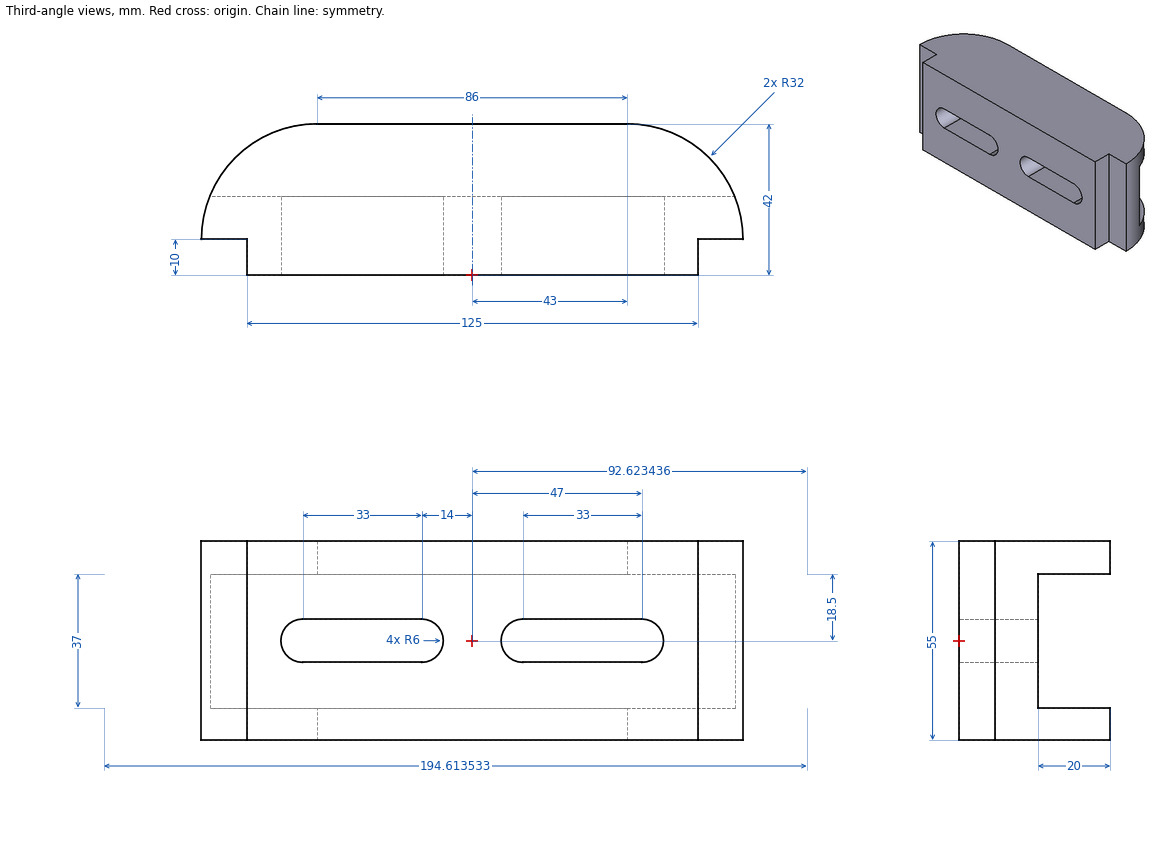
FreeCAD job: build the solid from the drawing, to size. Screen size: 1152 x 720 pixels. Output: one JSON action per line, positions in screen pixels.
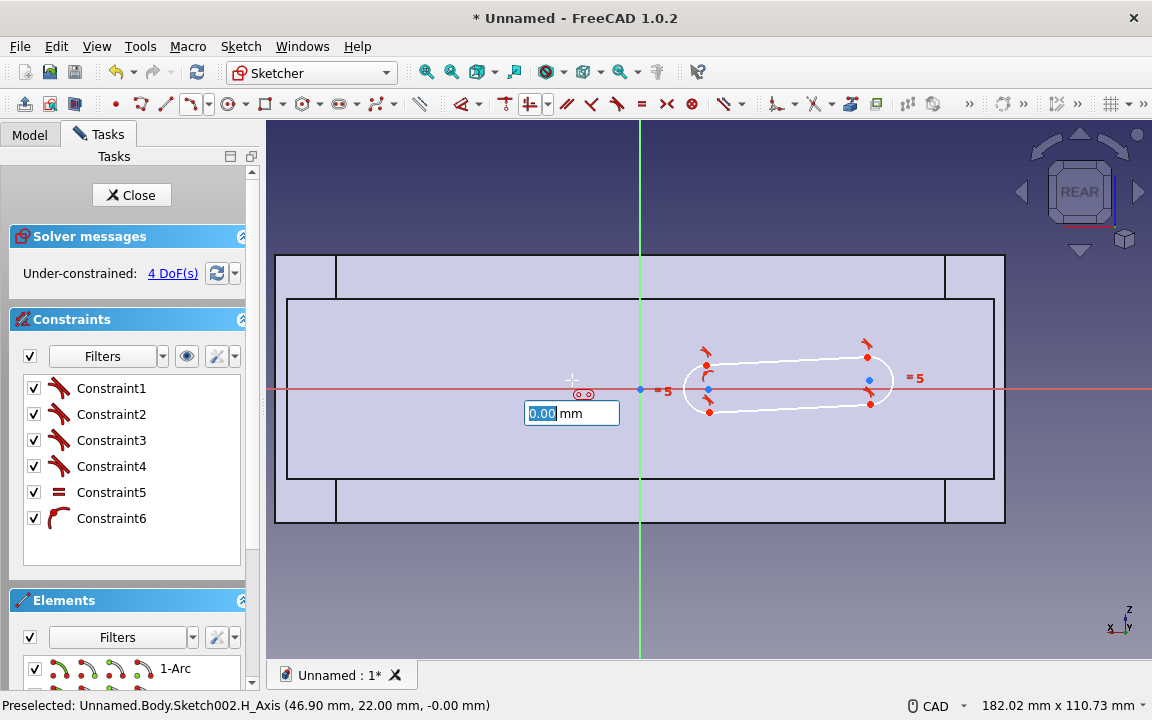
{"action": "left_click", "coordinate": [492, 418]}
{"action": "key", "text": "Escape"}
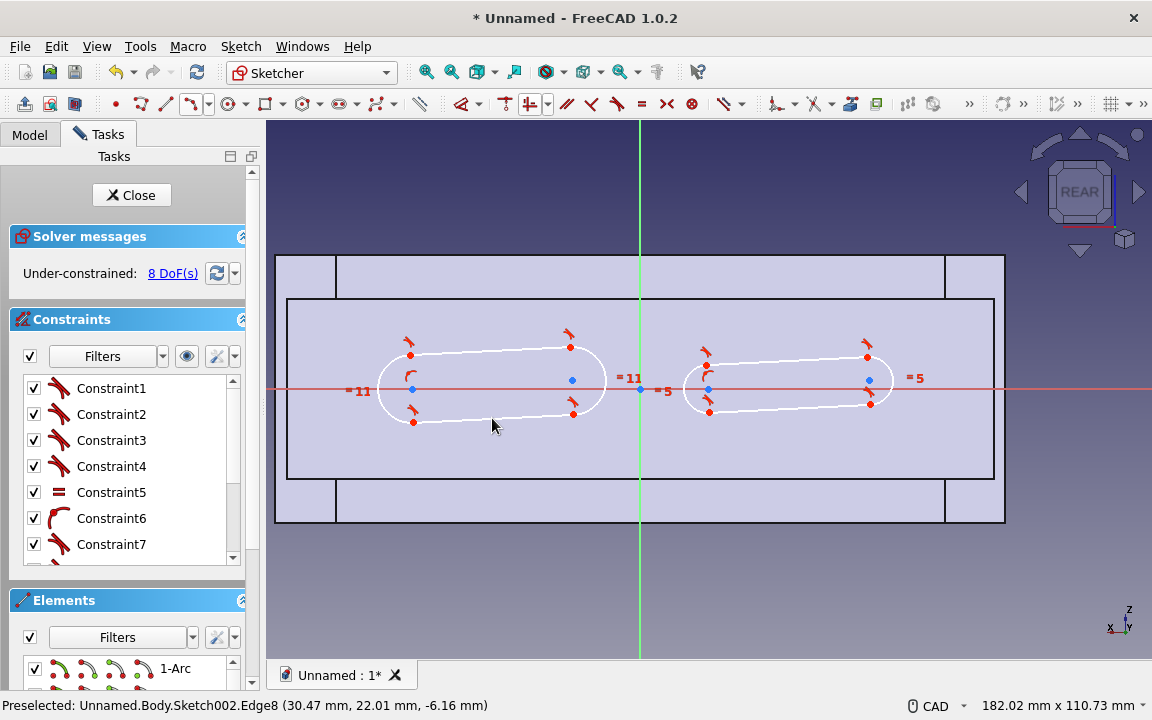
{"action": "left_click", "coordinate": [755, 363]}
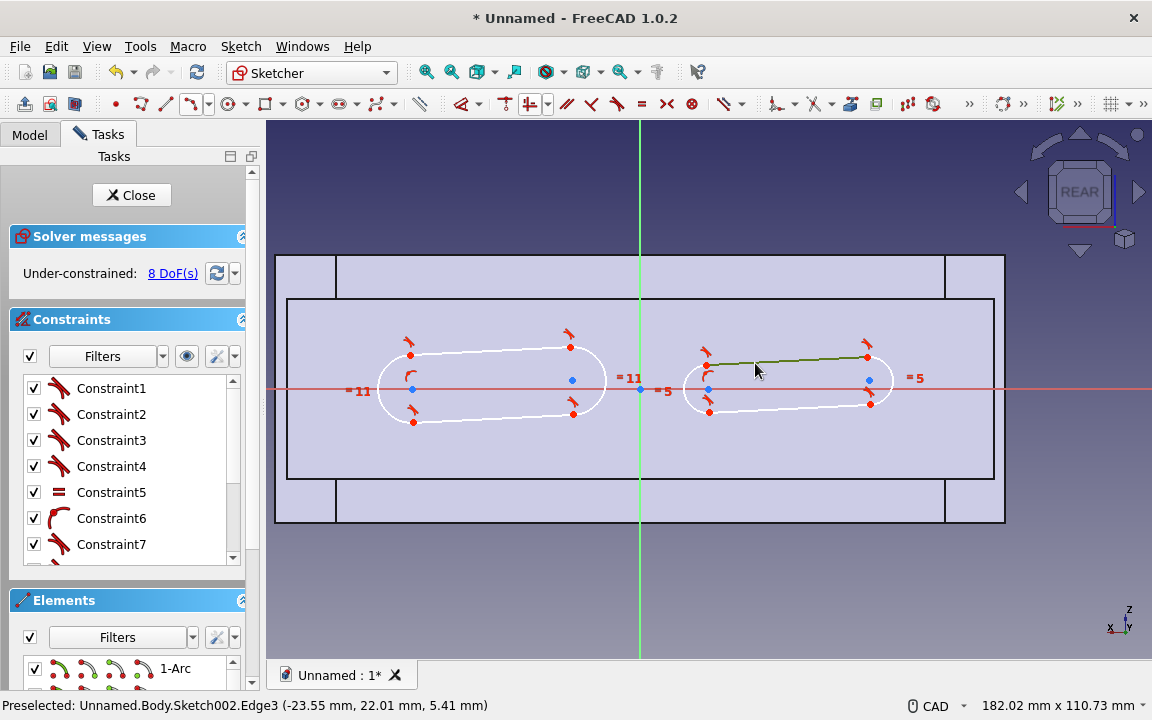
{"action": "key", "text": "h"}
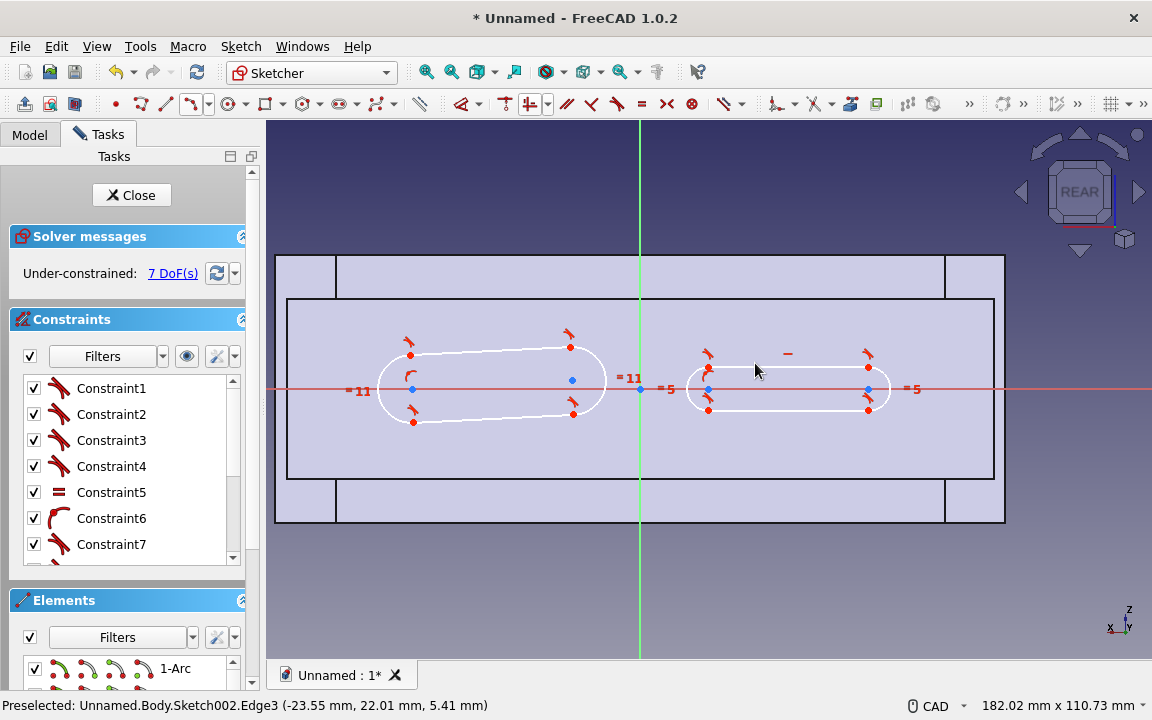
{"action": "left_click", "coordinate": [458, 353]}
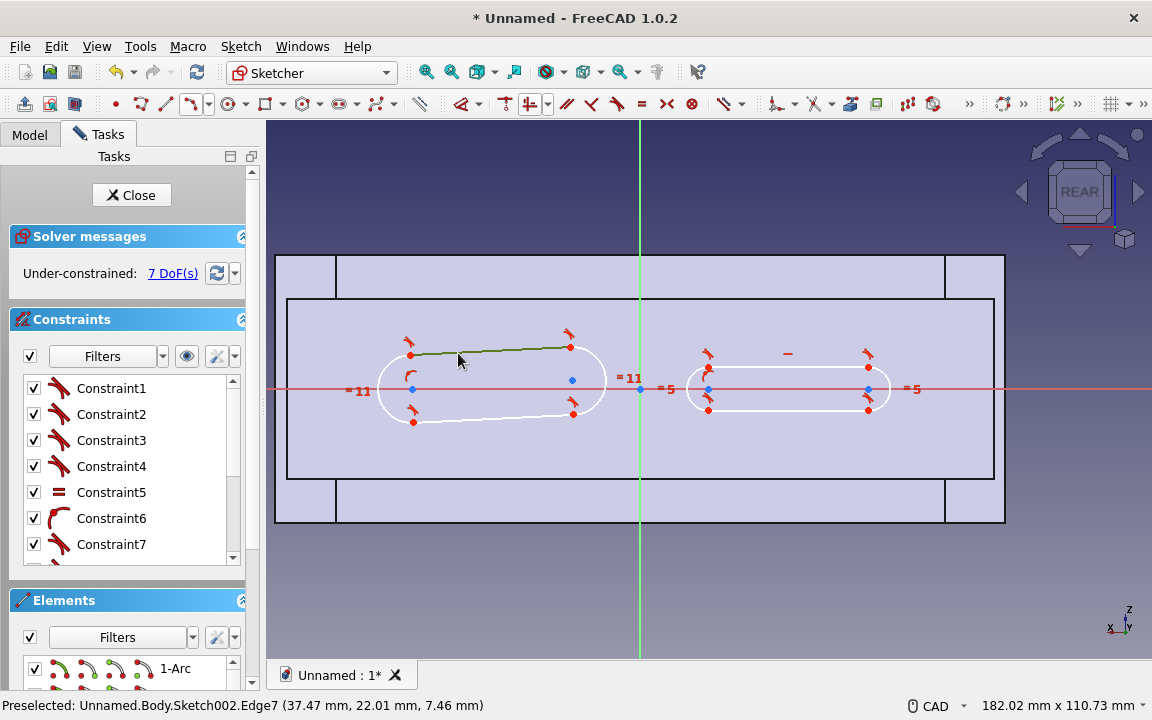
{"action": "left_click", "coordinate": [548, 104]}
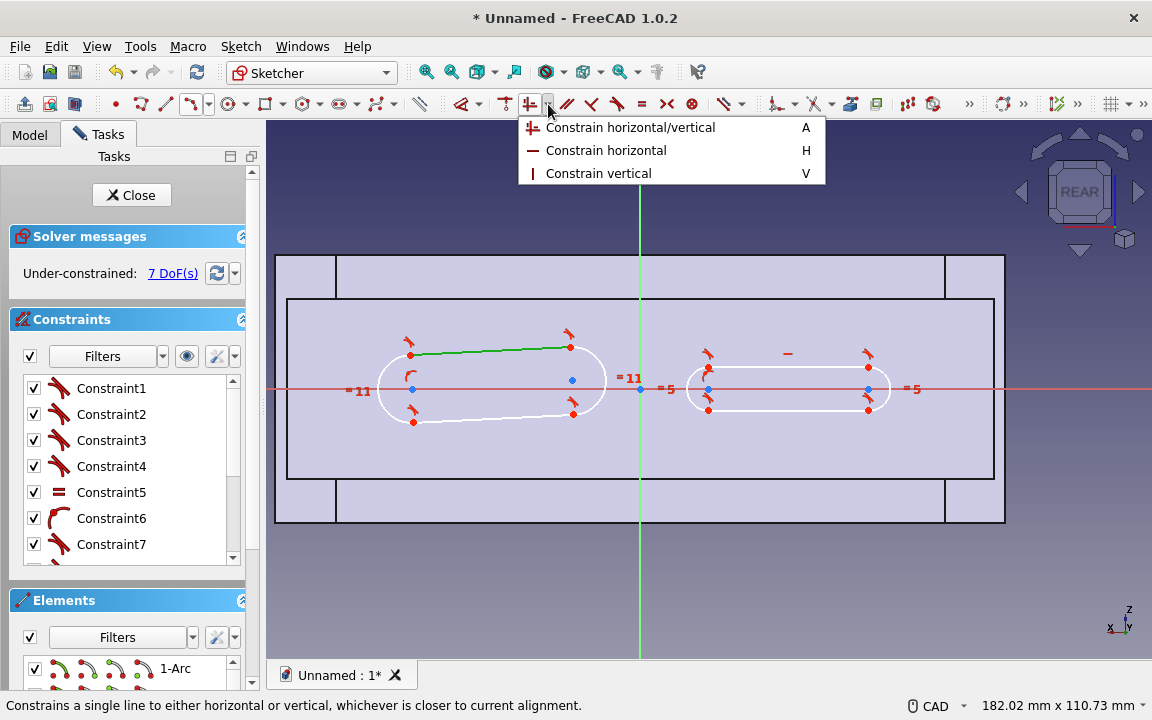
{"action": "left_click", "coordinate": [672, 150]}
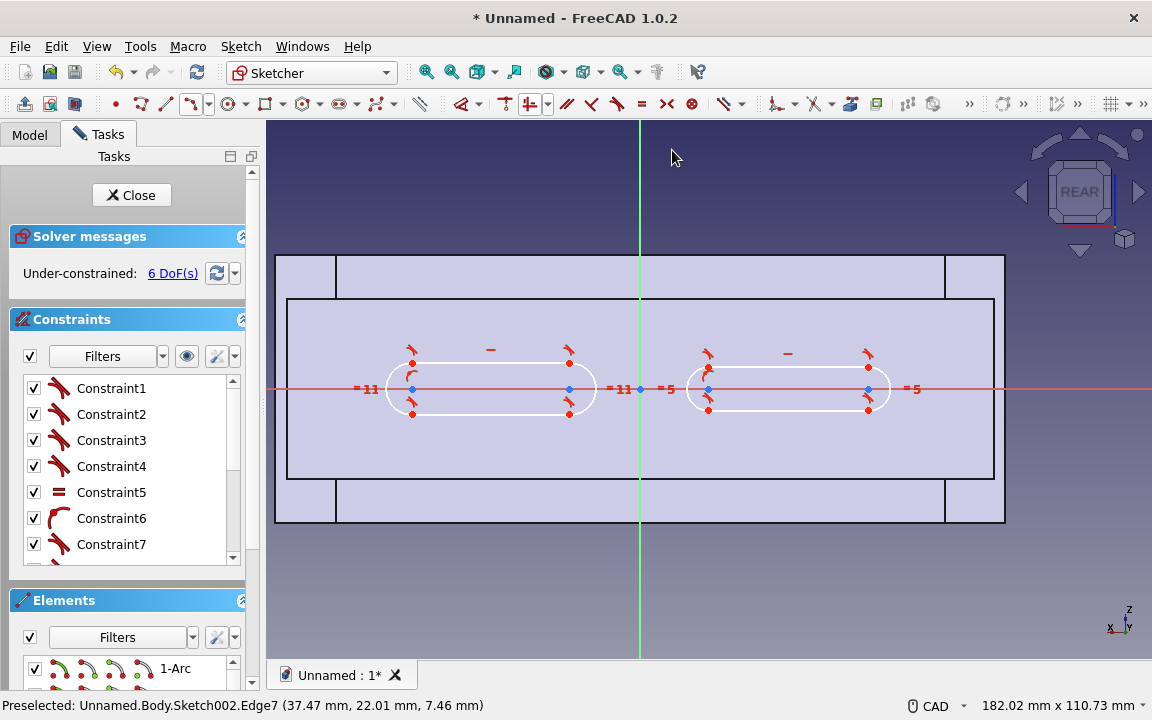
{"action": "left_click", "coordinate": [691, 376]}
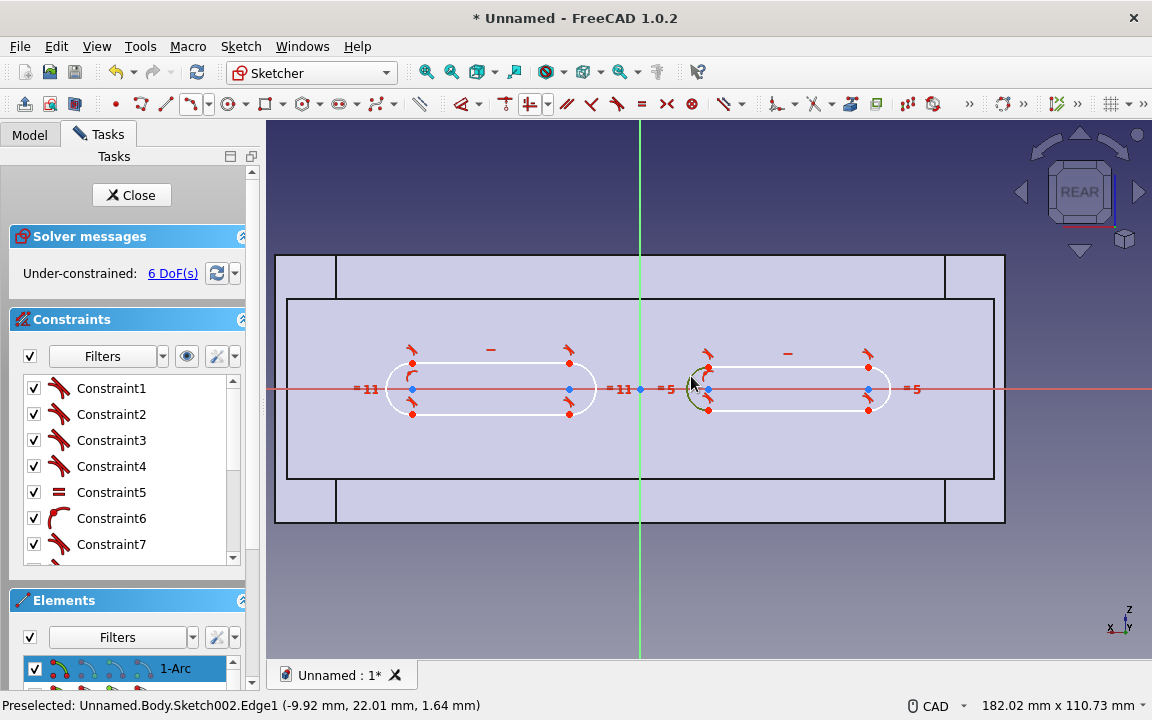
{"action": "left_click", "coordinate": [391, 374]}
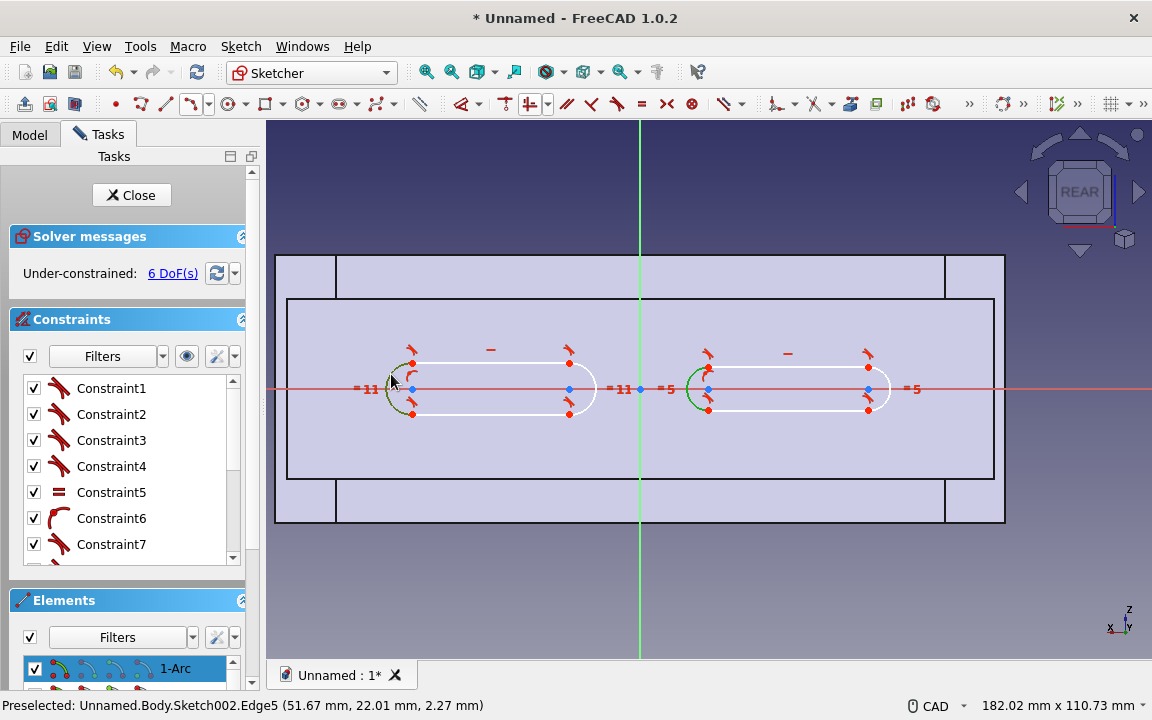
{"action": "left_click", "coordinate": [642, 104]}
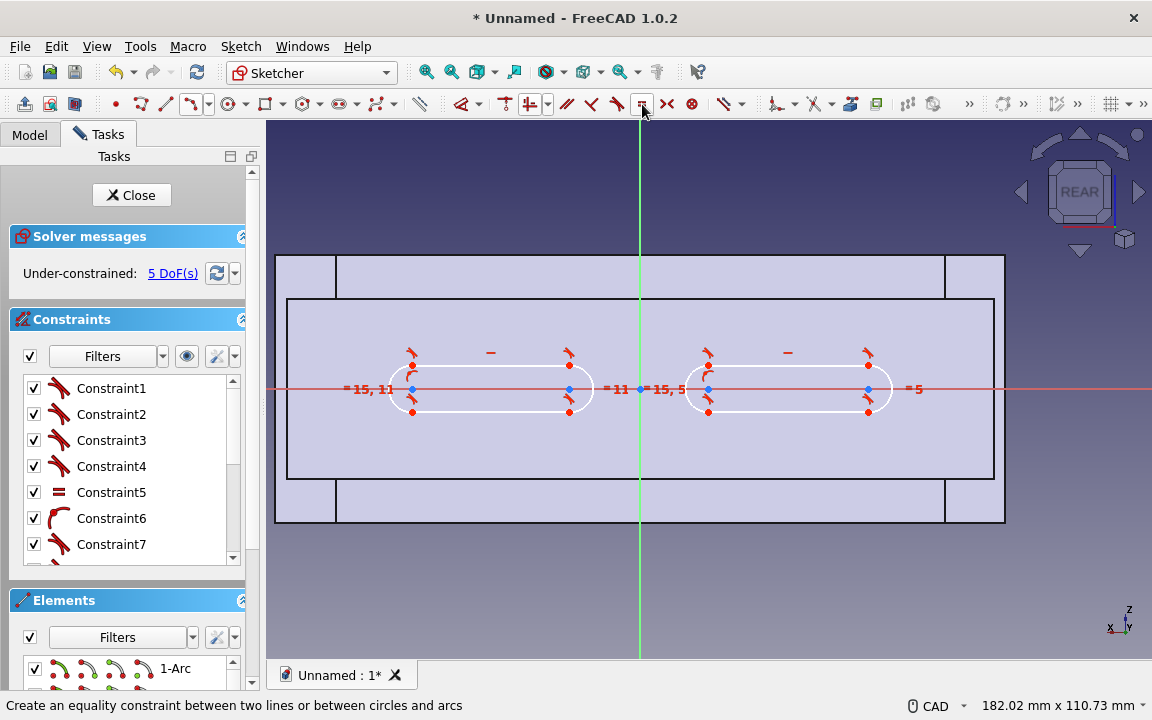
{"action": "left_click", "coordinate": [460, 104]}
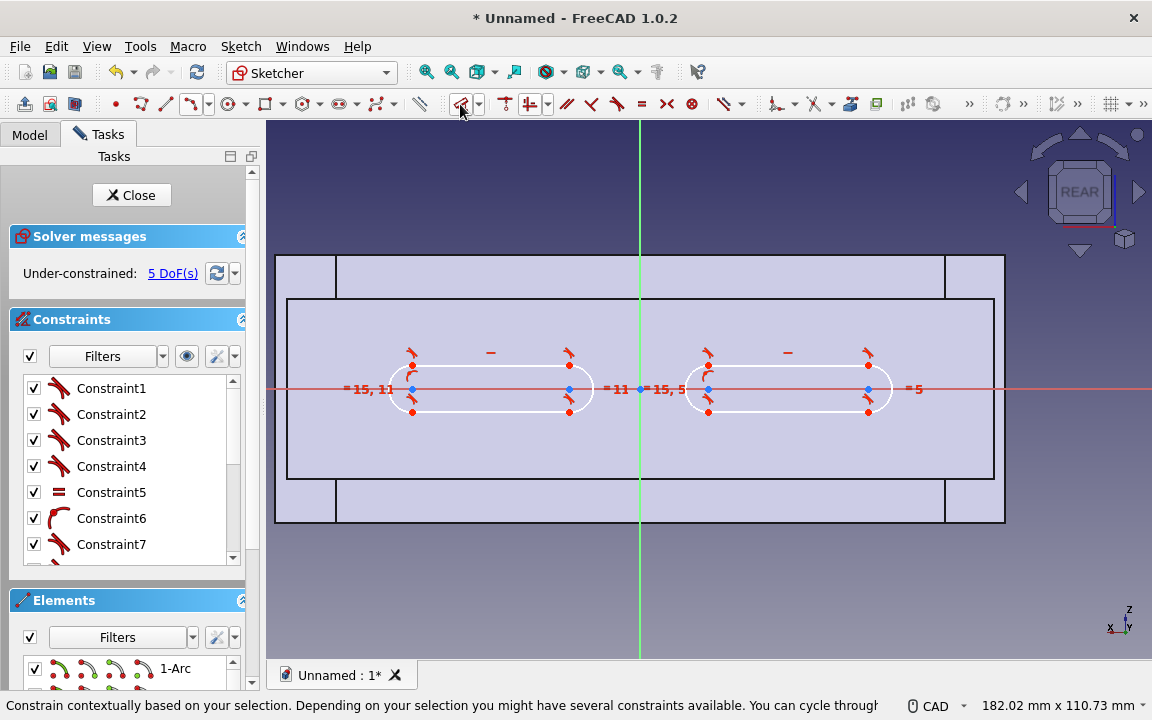
{"action": "scroll", "coordinate": [690, 375], "scroll_direction": "up", "scroll_amount": 2}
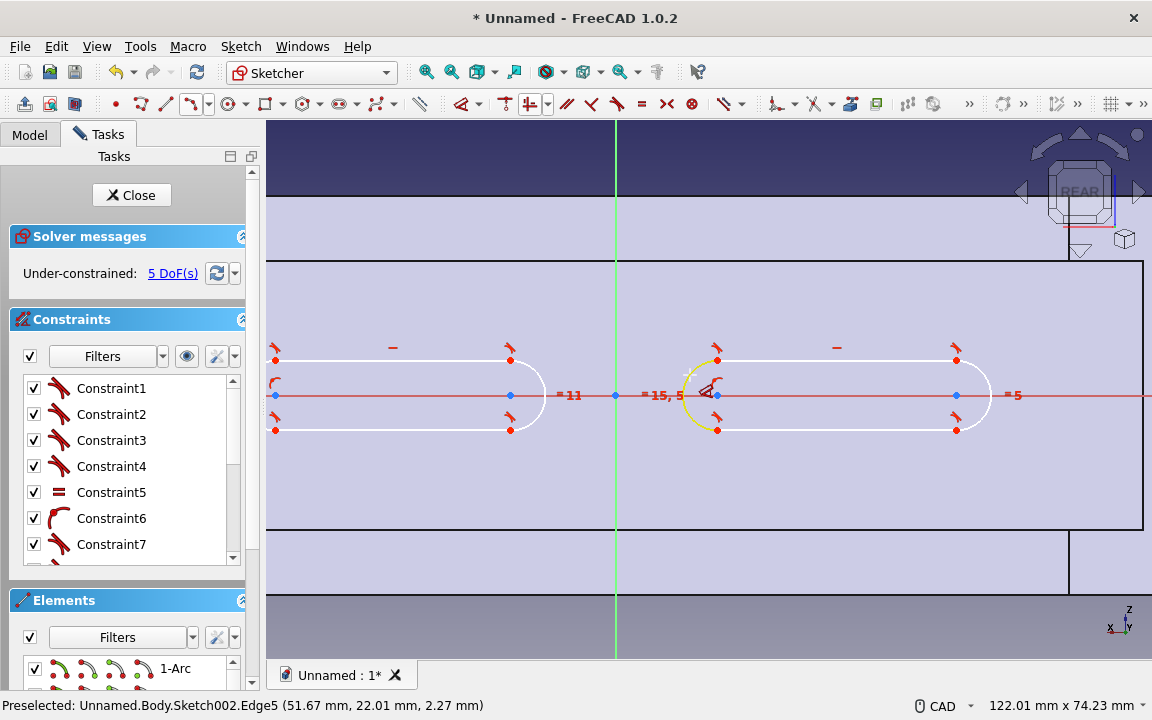
{"action": "left_click", "coordinate": [690, 375]}
{"action": "left_click", "coordinate": [664, 356]}